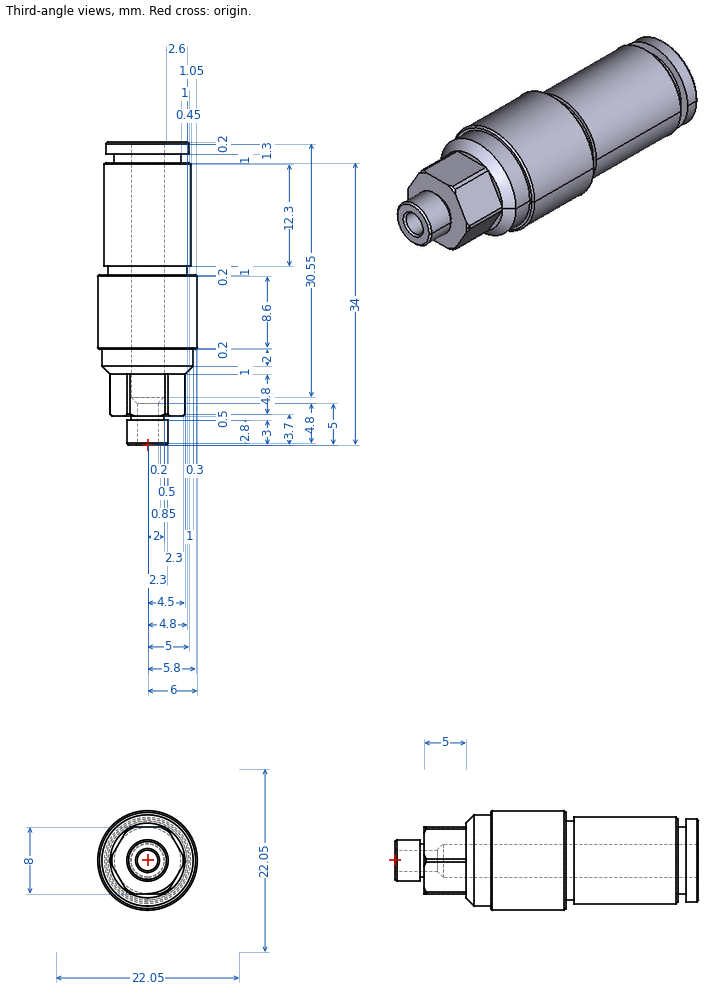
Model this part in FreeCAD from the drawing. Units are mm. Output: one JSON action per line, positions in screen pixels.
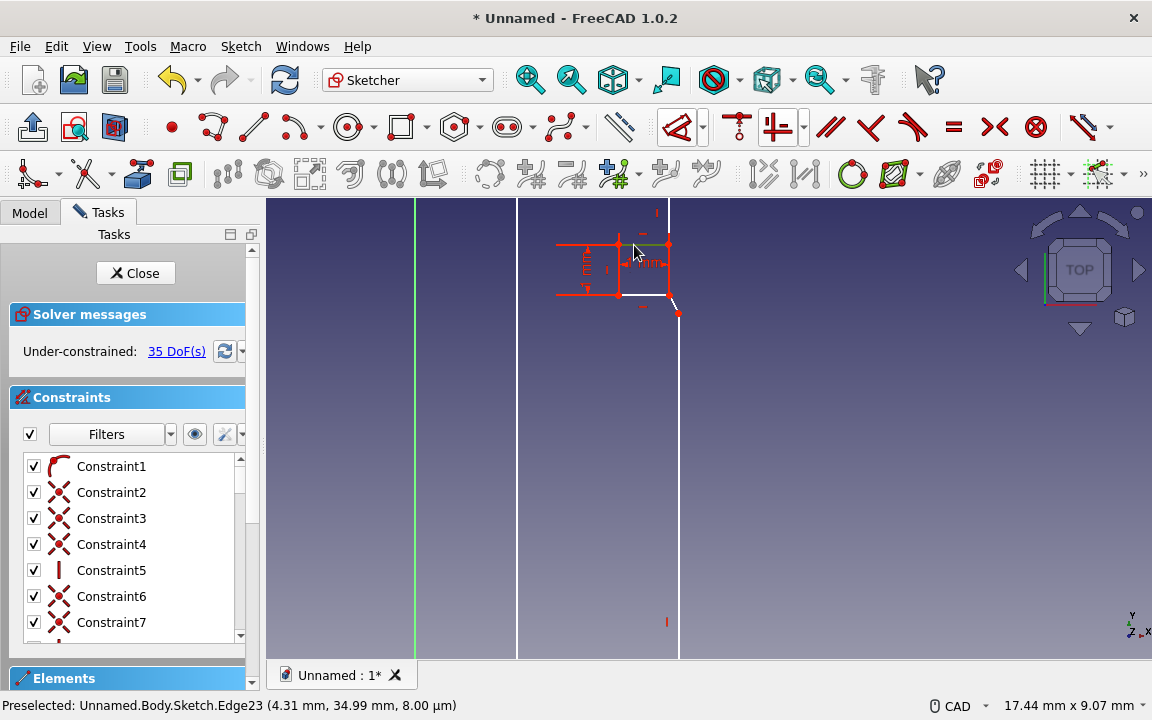
{"action": "left_click", "coordinate": [702, 128]}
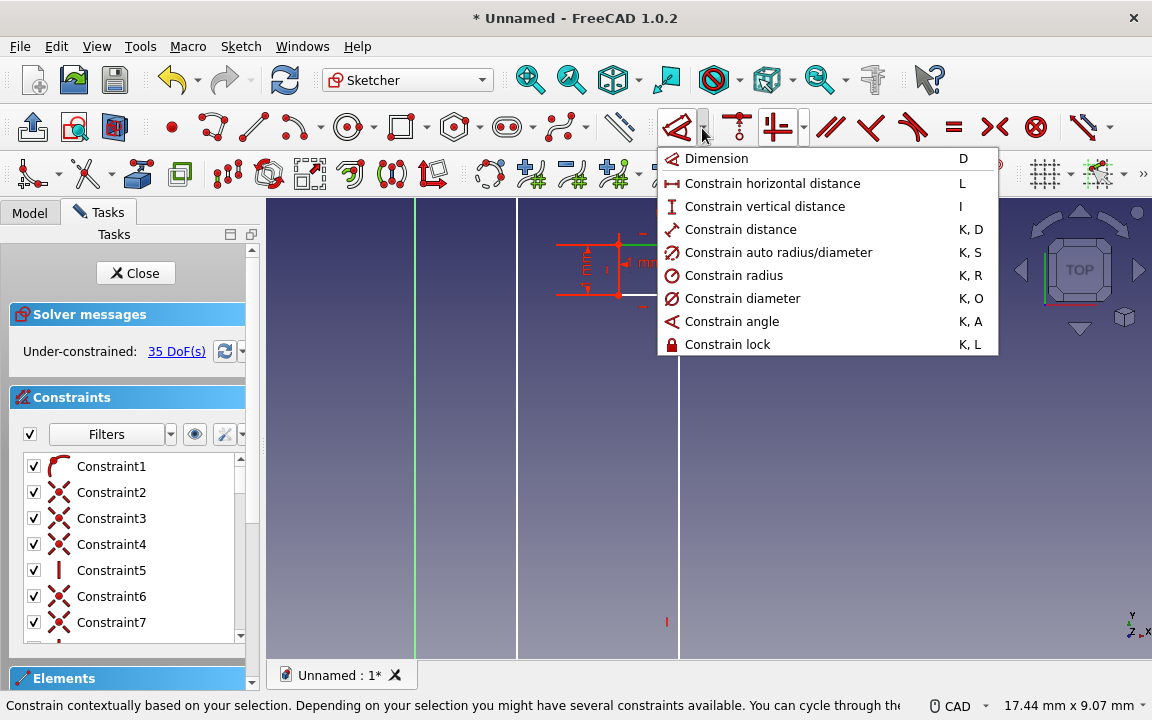
{"action": "left_click", "coordinate": [828, 184]}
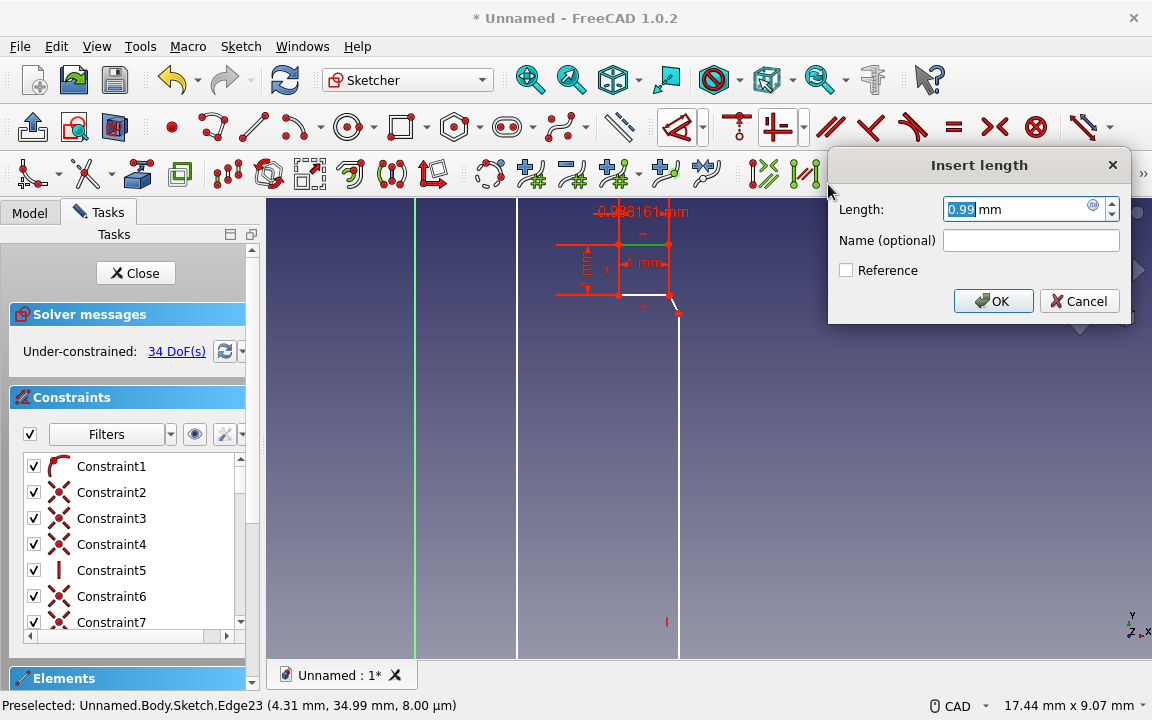
{"action": "type", "text": "1"}
{"action": "key", "text": "Return"}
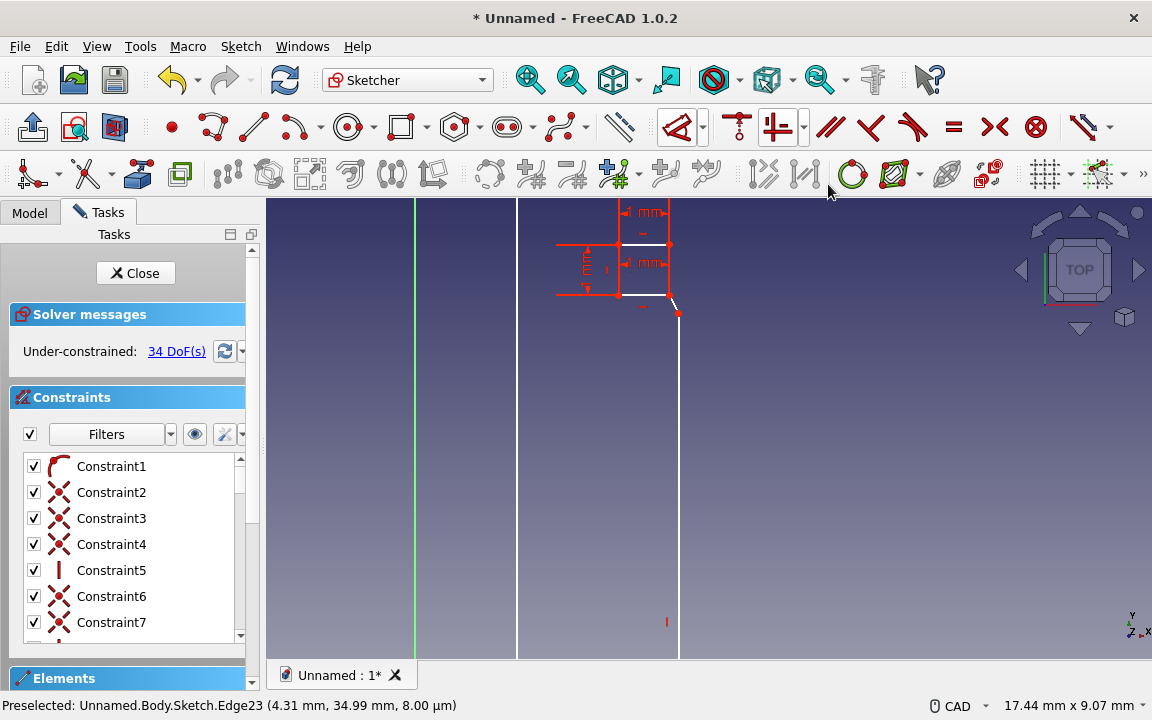
{"action": "scroll", "coordinate": [655, 297], "scroll_direction": "down", "scroll_amount": 9}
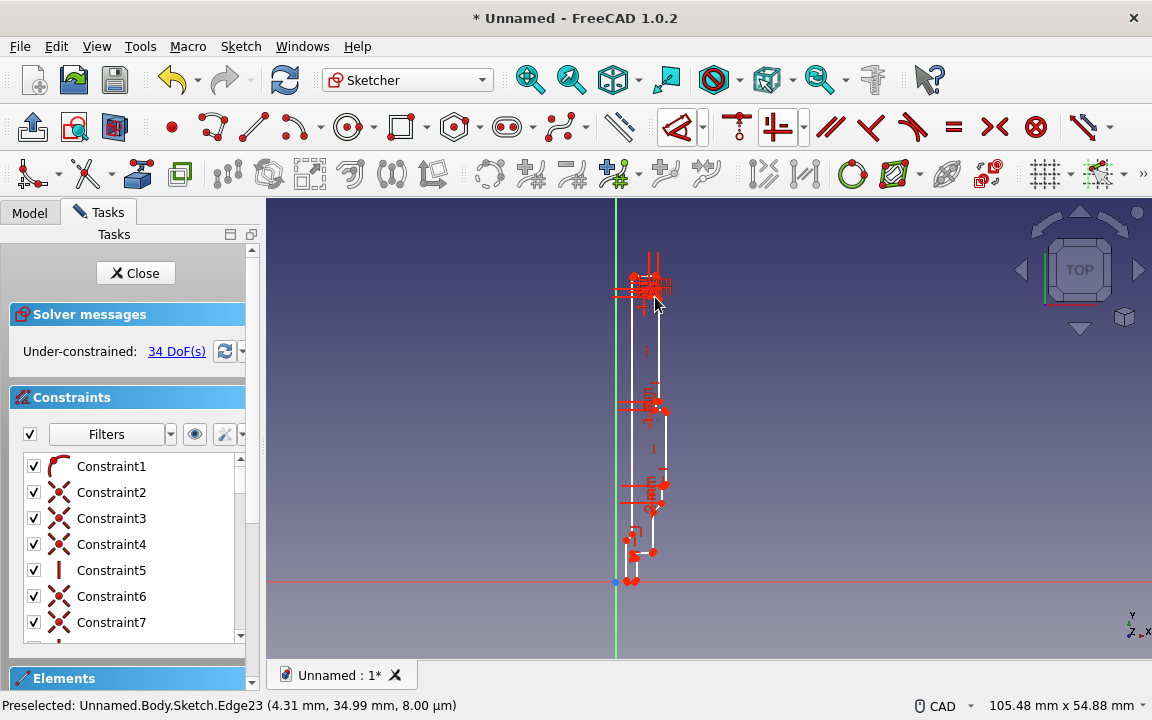
{"action": "scroll", "coordinate": [637, 558], "scroll_direction": "up", "scroll_amount": 6}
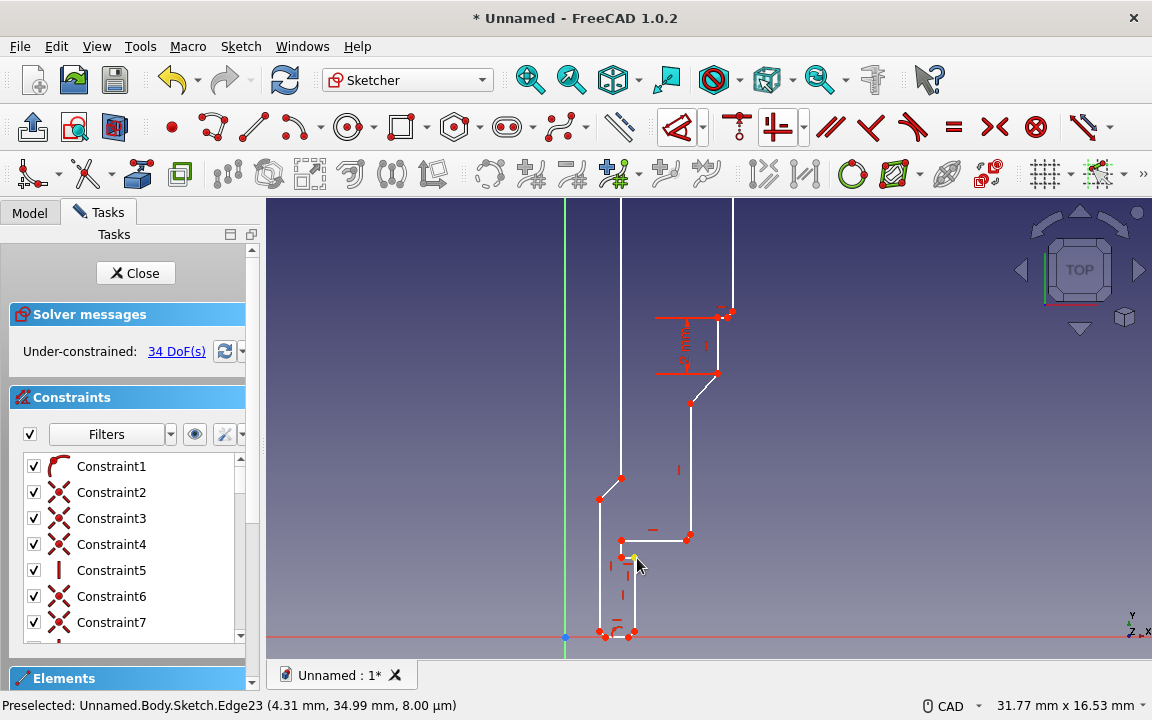
{"action": "left_click", "coordinate": [635, 558]}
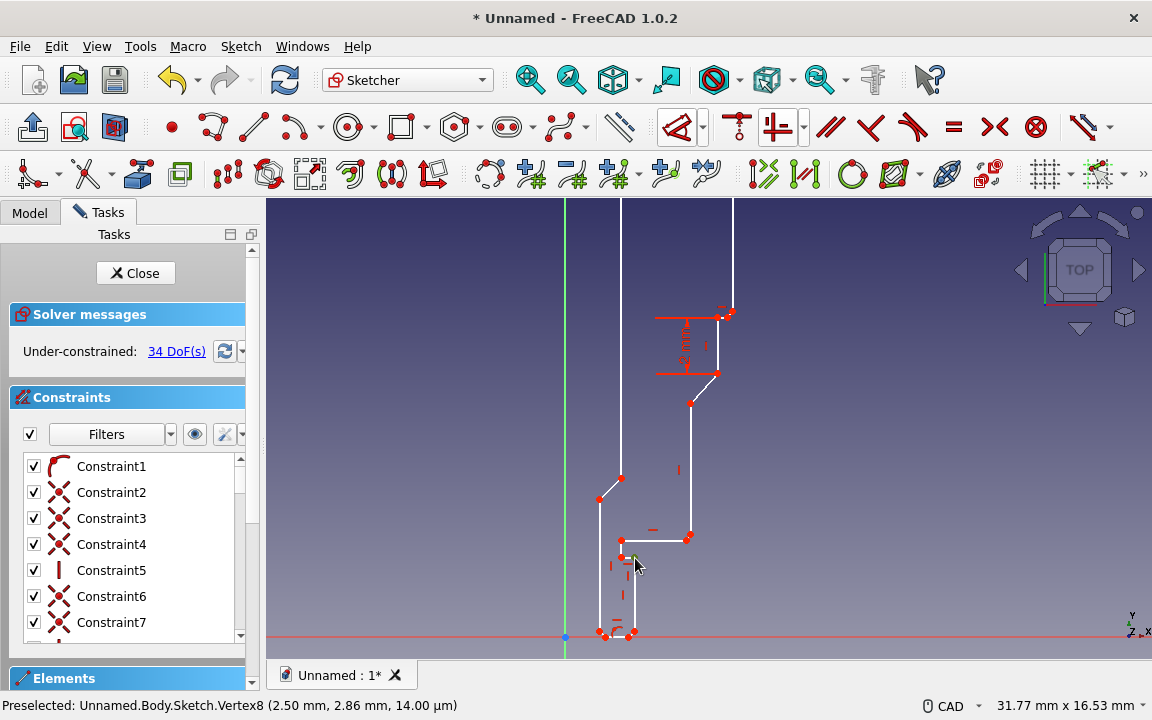
{"action": "key", "text": "i"}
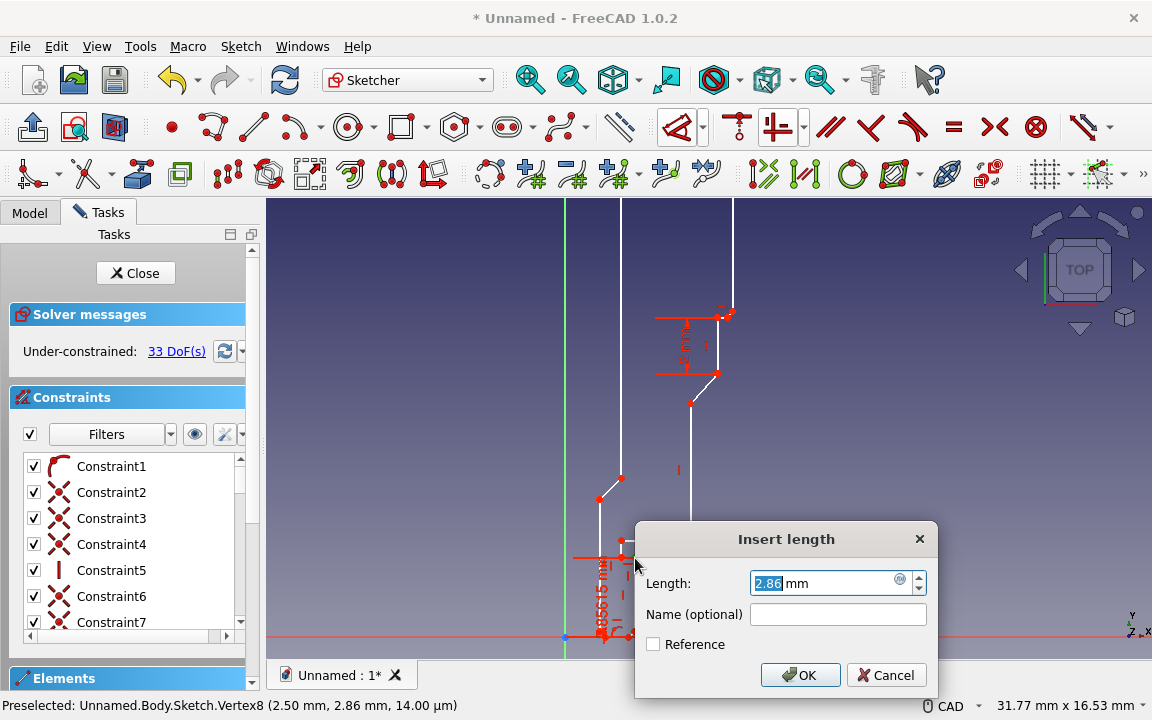
{"action": "type", "text": "3"}
{"action": "key", "text": "Return"}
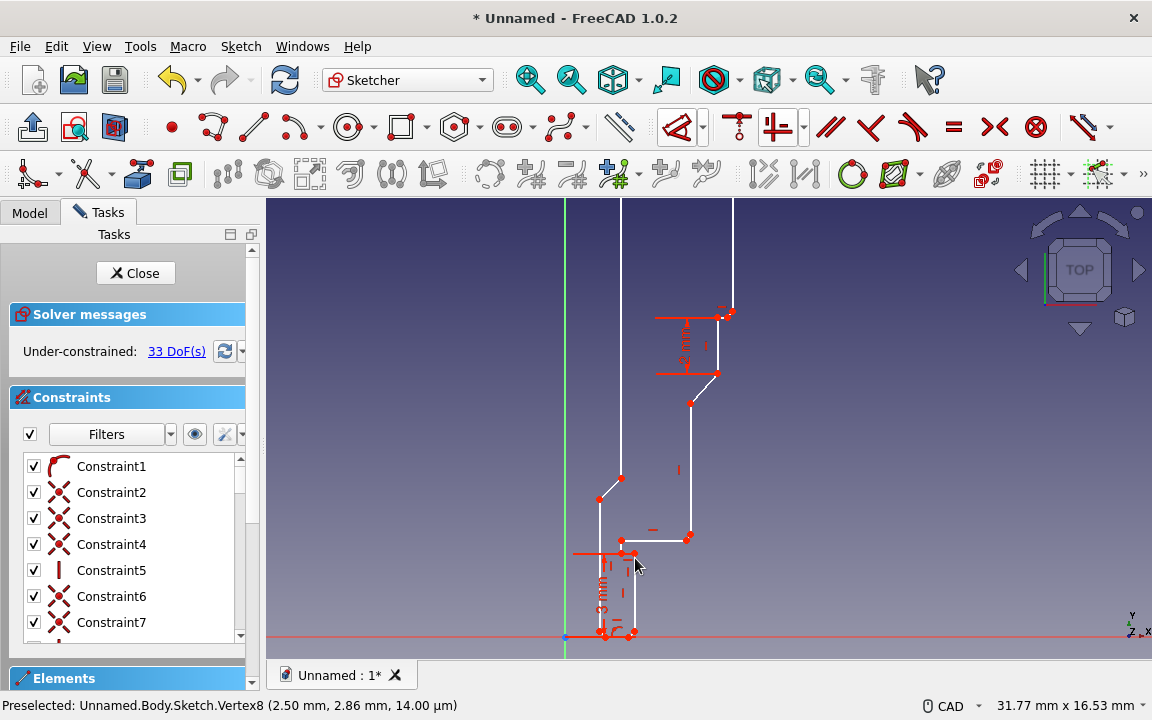
{"action": "left_click", "coordinate": [621, 554]}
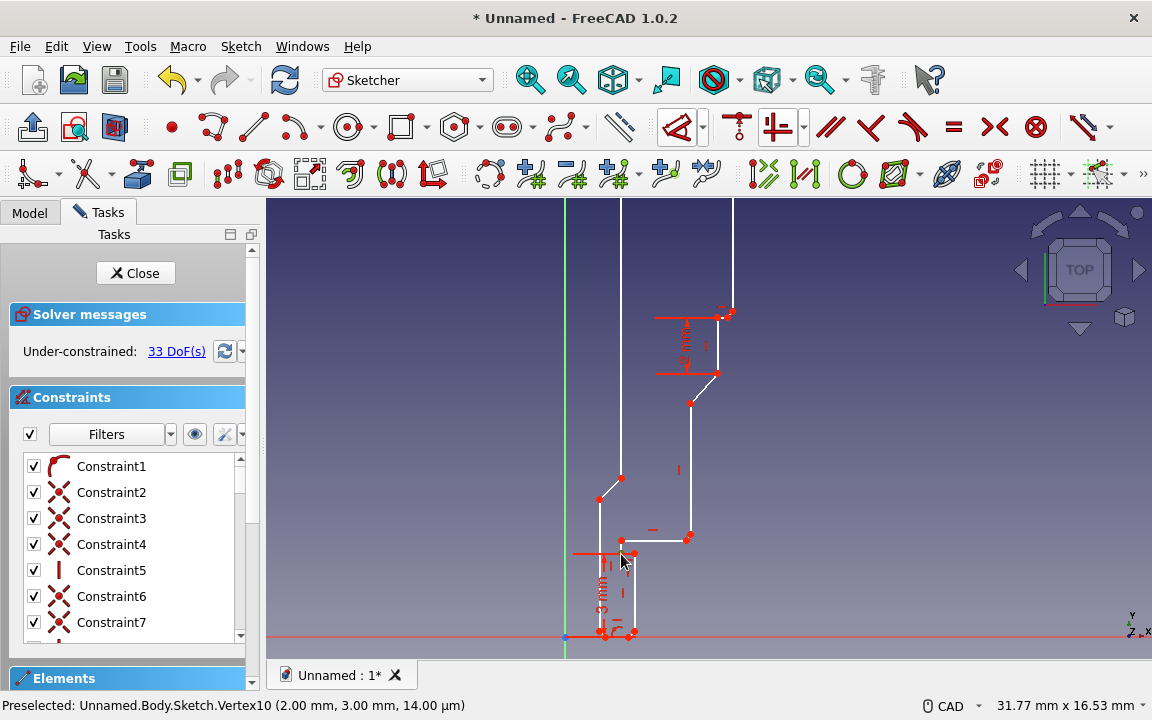
{"action": "key", "text": "l"}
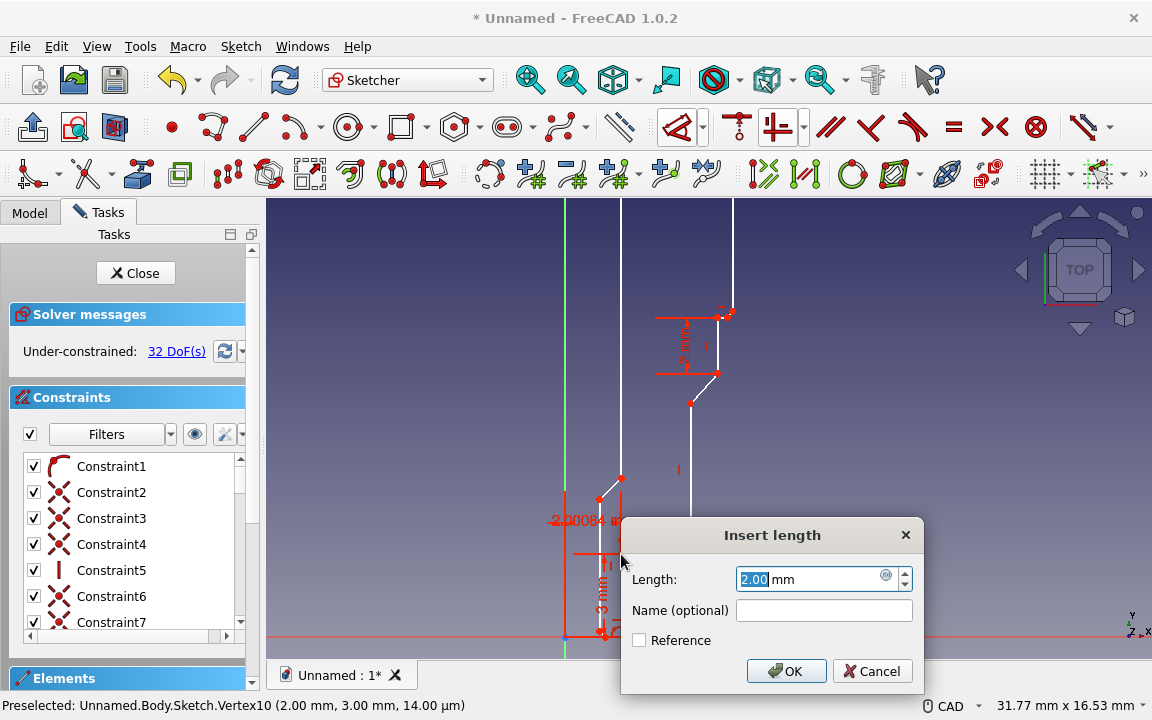
{"action": "type", "text": "2"}
{"action": "key", "text": "Return"}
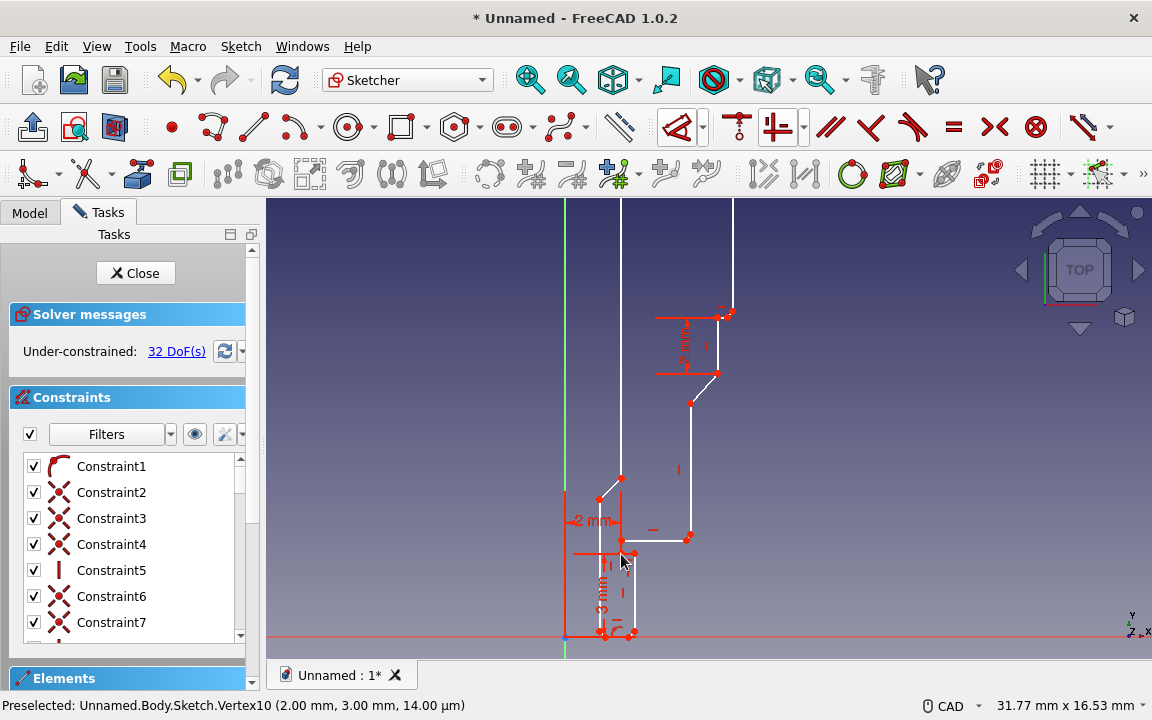
{"action": "scroll", "coordinate": [733, 311], "scroll_direction": "up", "scroll_amount": 2}